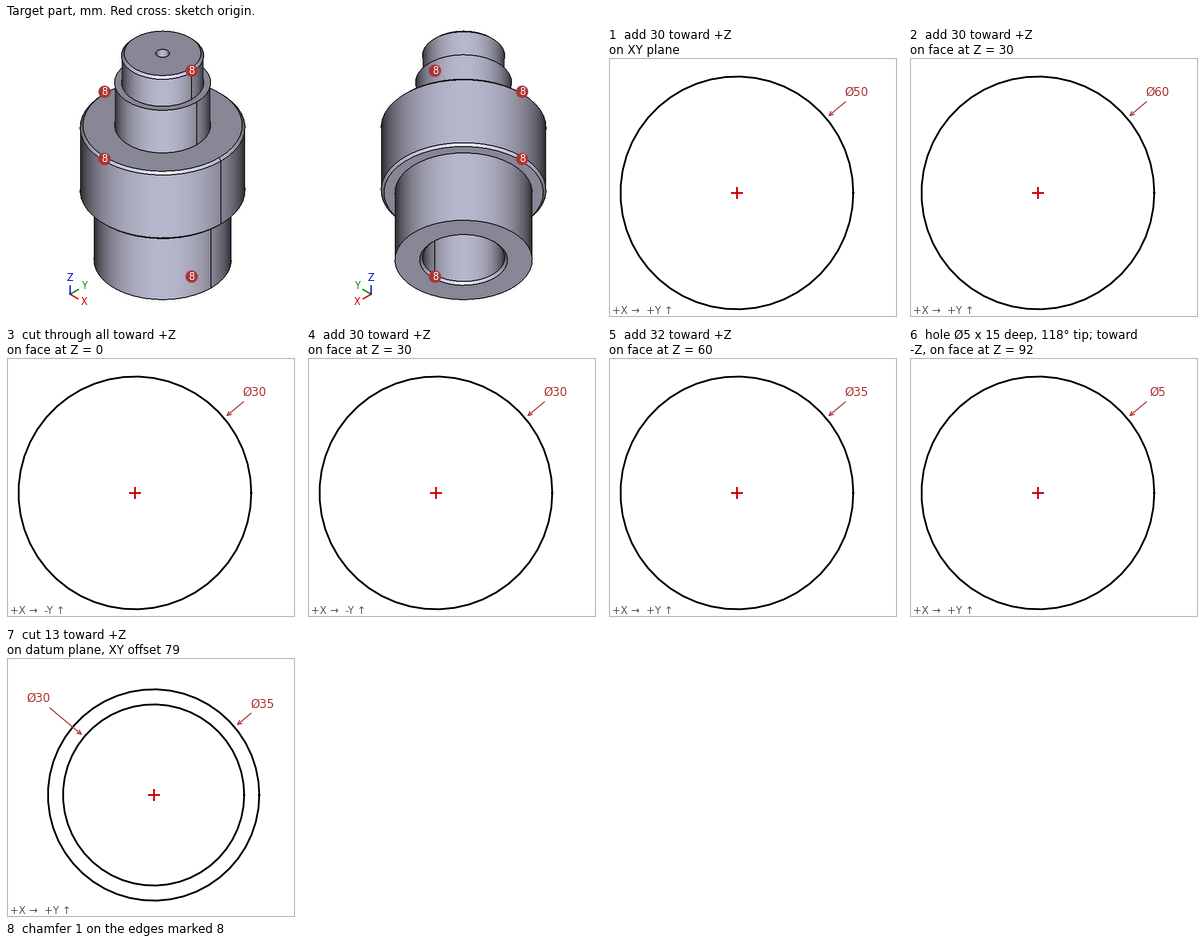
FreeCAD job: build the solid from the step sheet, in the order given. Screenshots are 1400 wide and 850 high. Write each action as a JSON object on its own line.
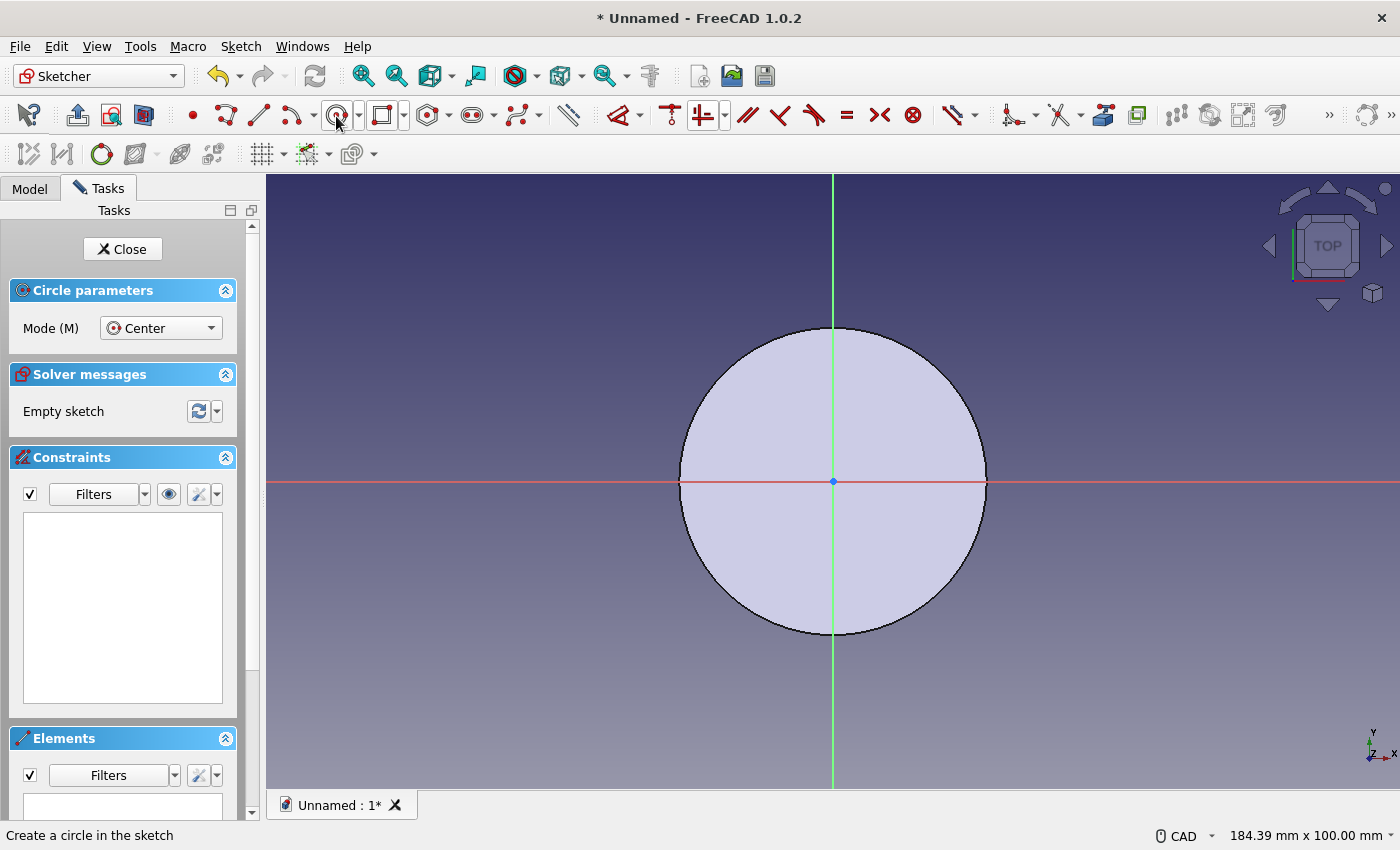
{"action": "left_click", "coordinate": [833, 482]}
{"action": "left_click", "coordinate": [963, 351]}
{"action": "key", "text": "Escape"}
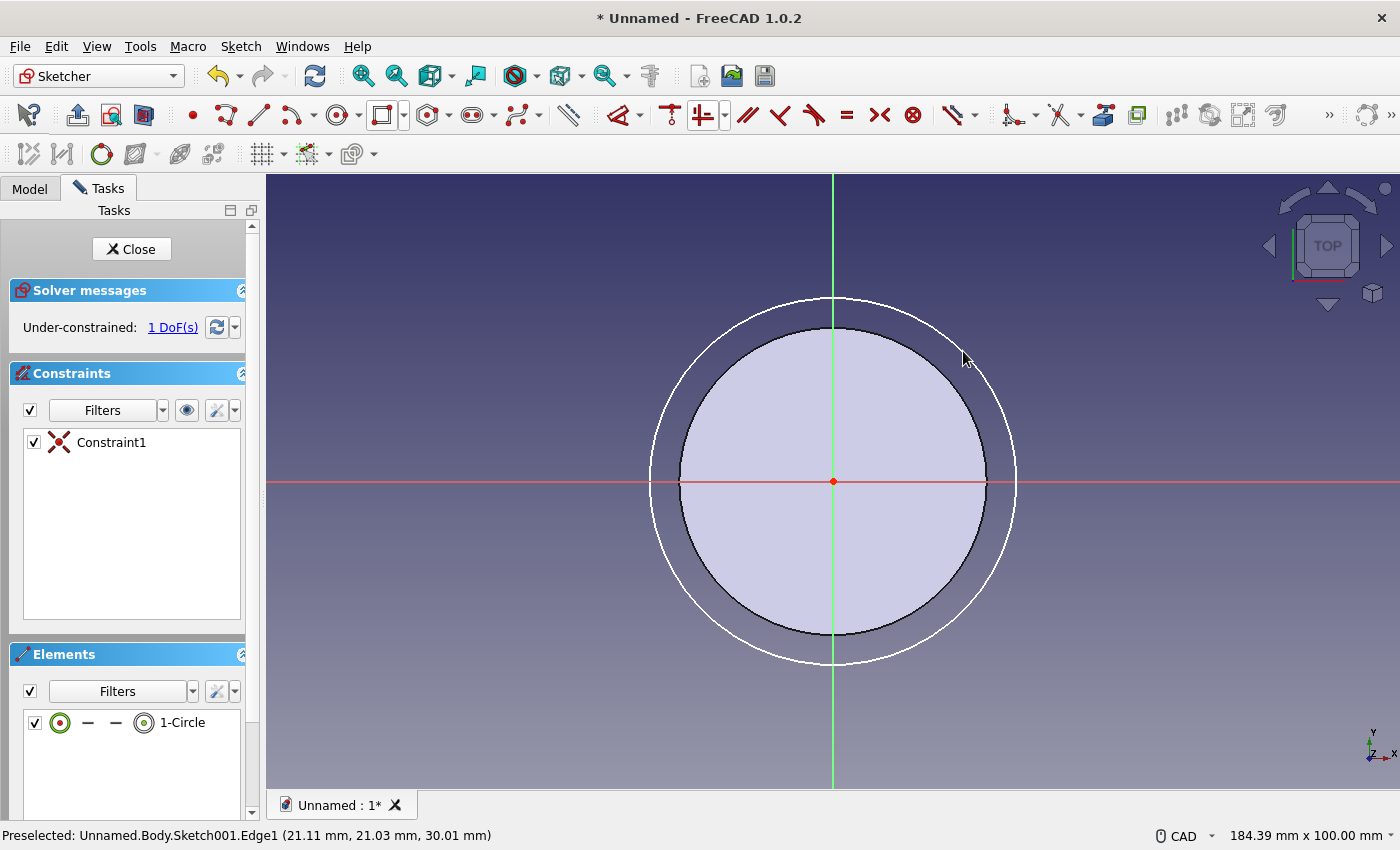
{"action": "key", "text": "d"}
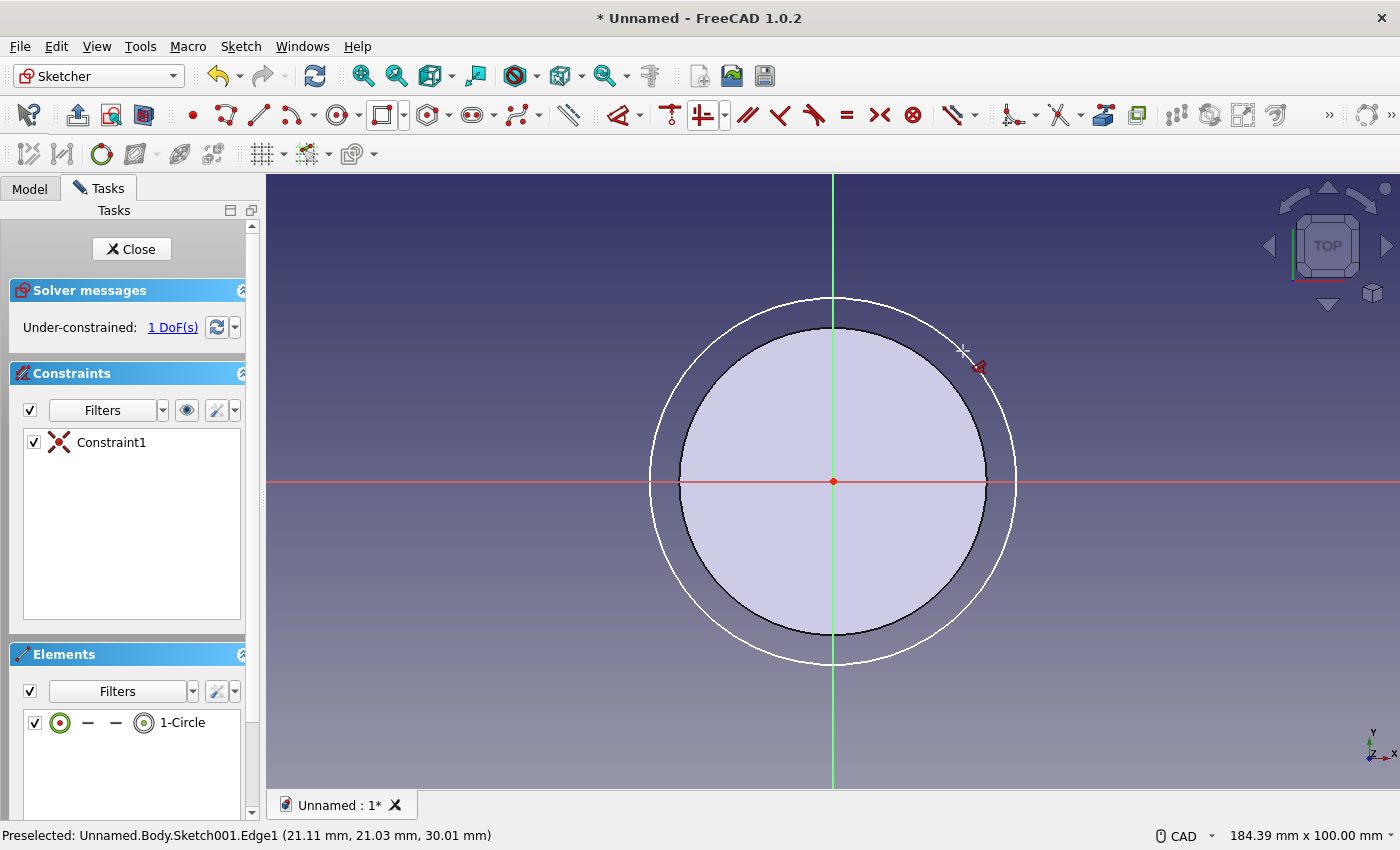
{"action": "left_click", "coordinate": [962, 351]}
{"action": "left_click", "coordinate": [984, 328]}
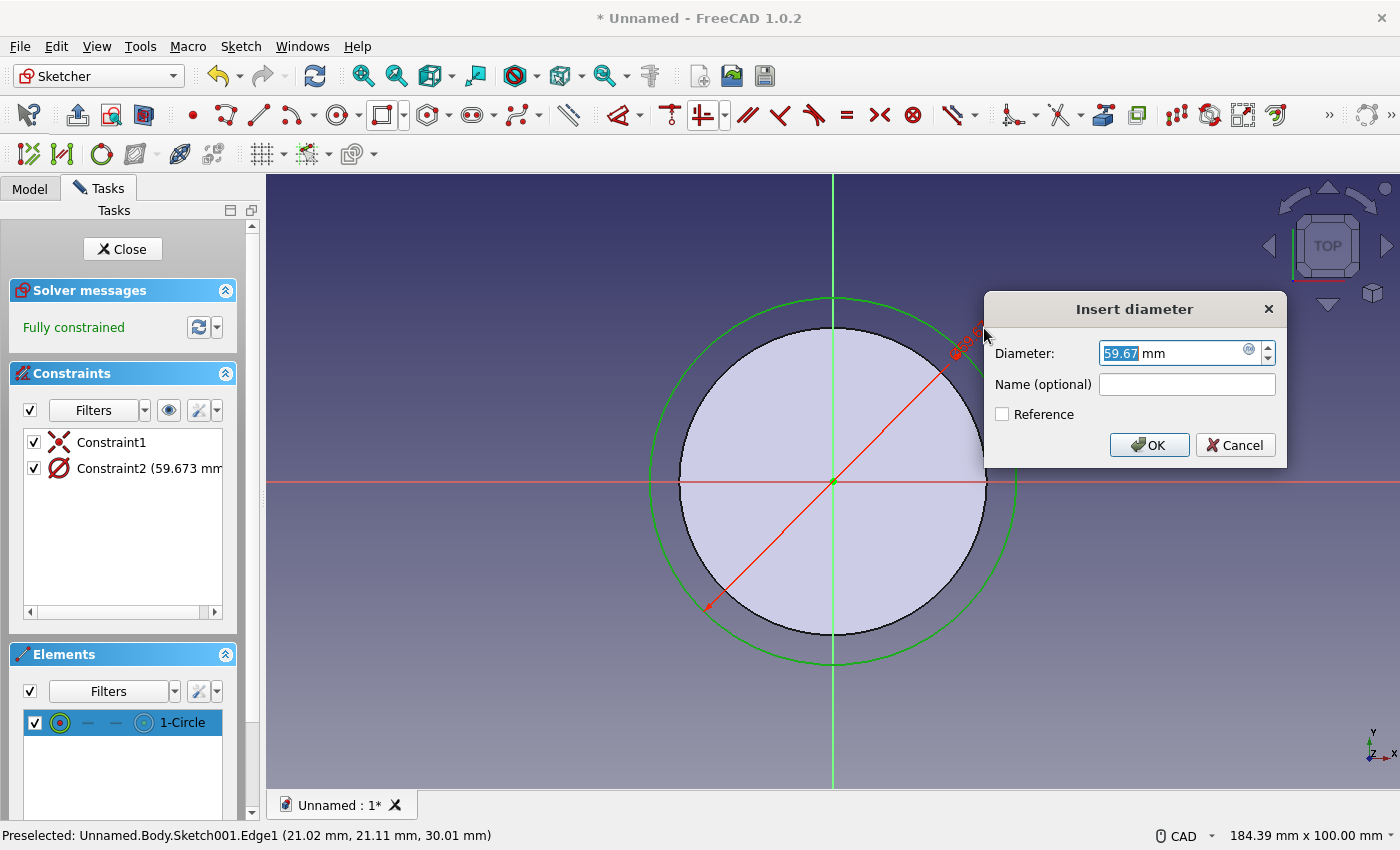
{"action": "type", "text": "60"}
{"action": "key", "text": "Return"}
{"action": "key", "text": "Escape"}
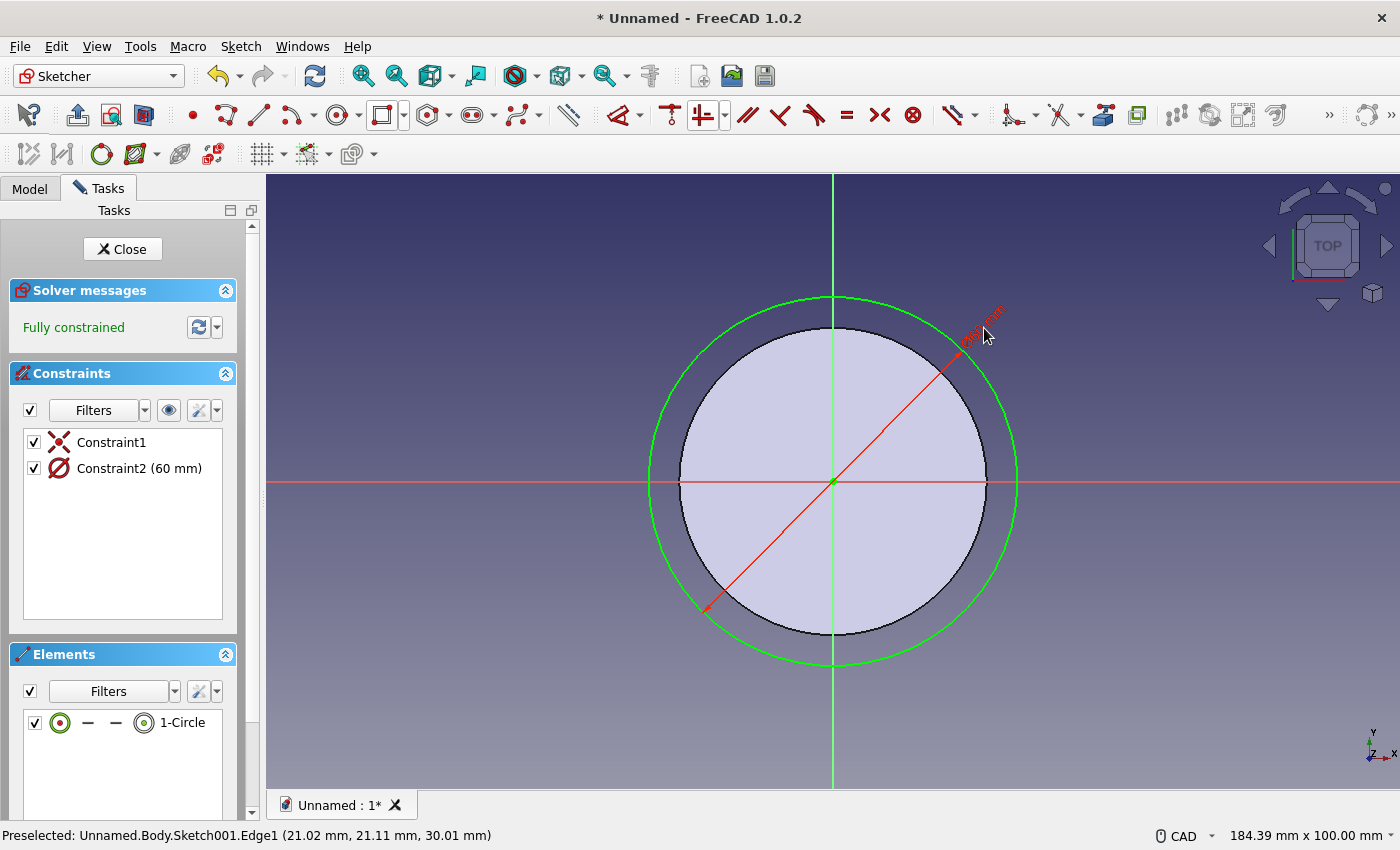
{"action": "left_click", "coordinate": [123, 249]}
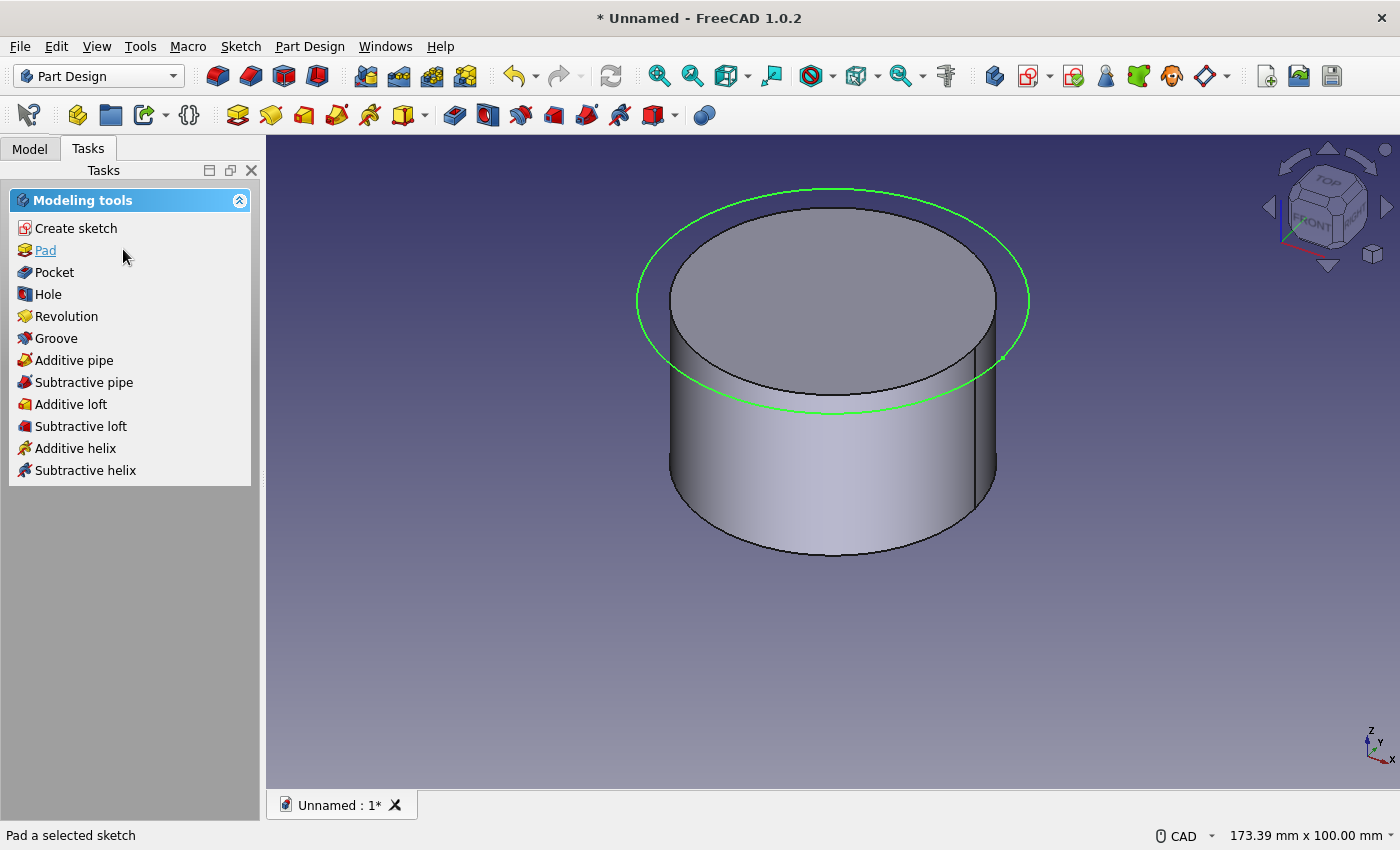
{"action": "left_click", "coordinate": [238, 116]}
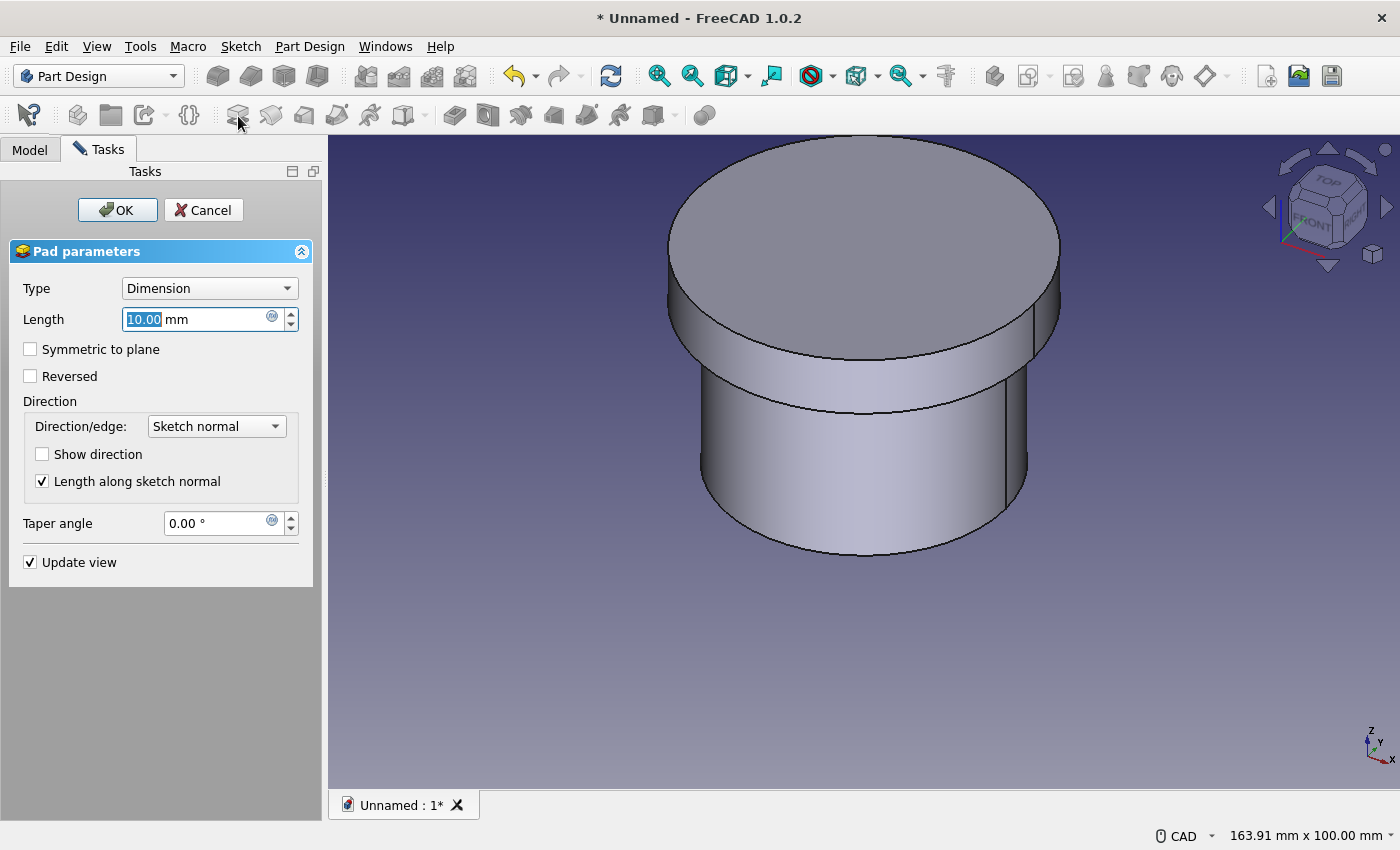
{"action": "type", "text": "30"}
{"action": "key", "text": "Tab"}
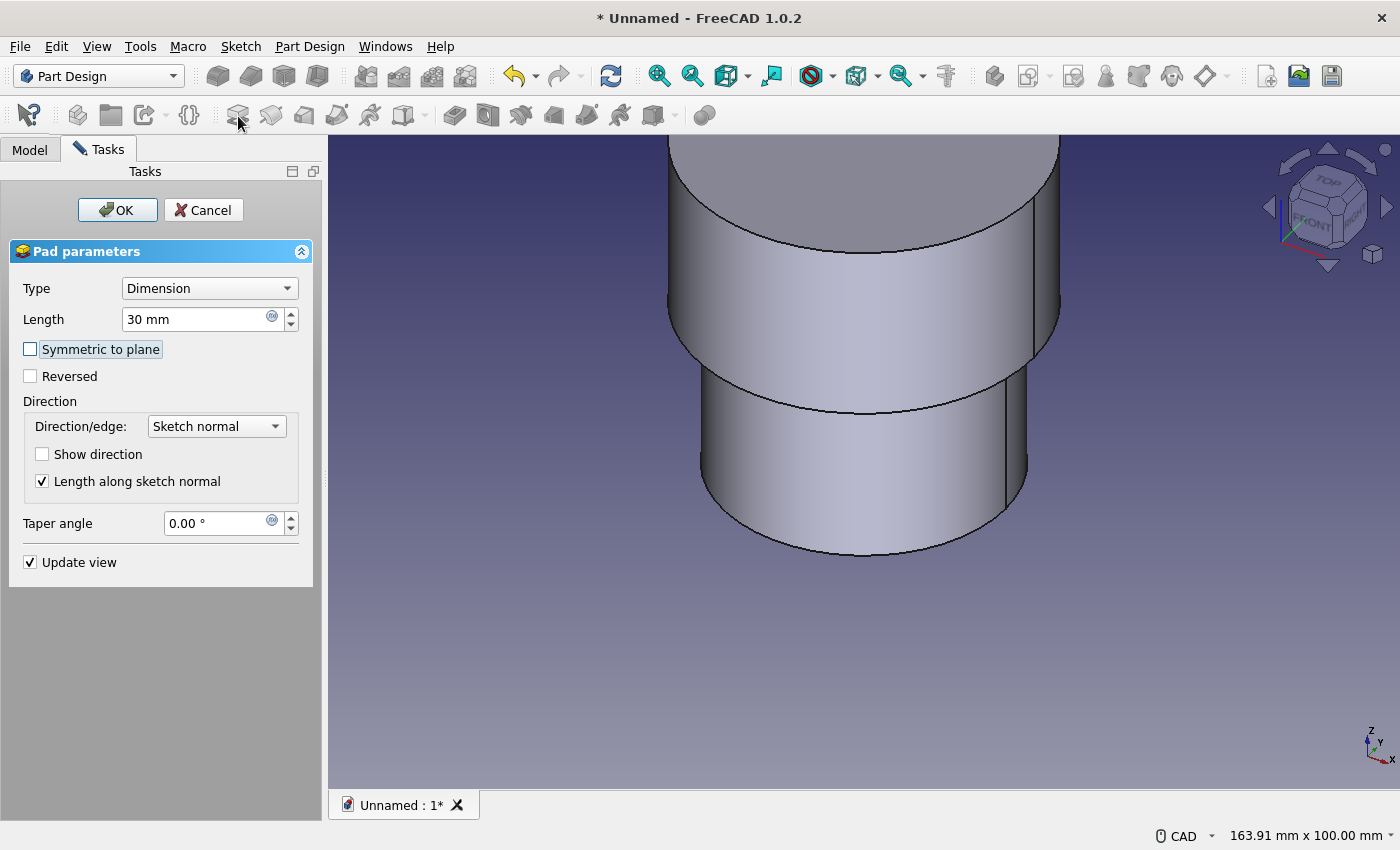
{"action": "left_click", "coordinate": [118, 210]}